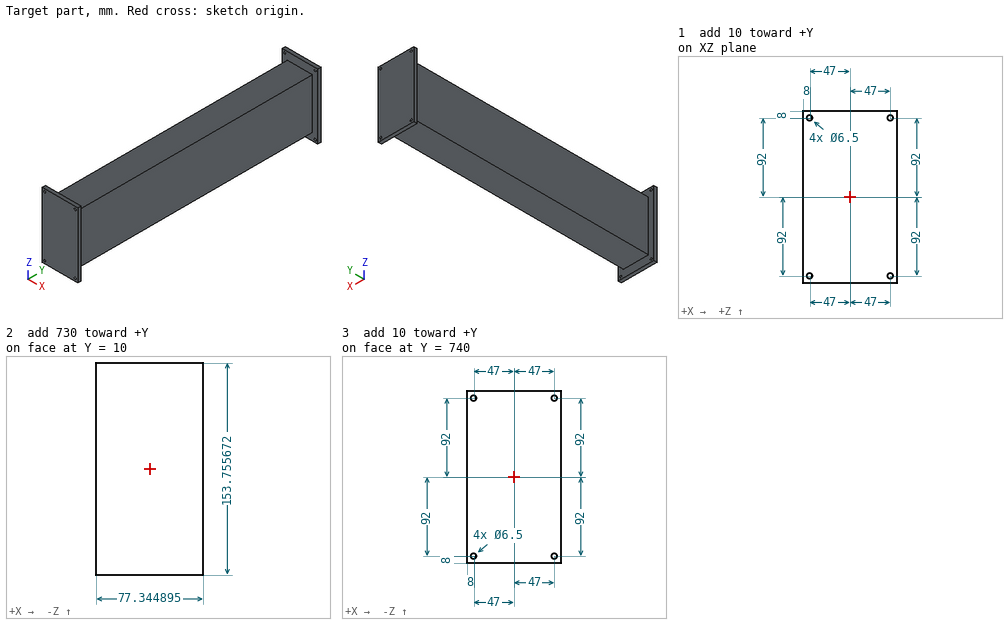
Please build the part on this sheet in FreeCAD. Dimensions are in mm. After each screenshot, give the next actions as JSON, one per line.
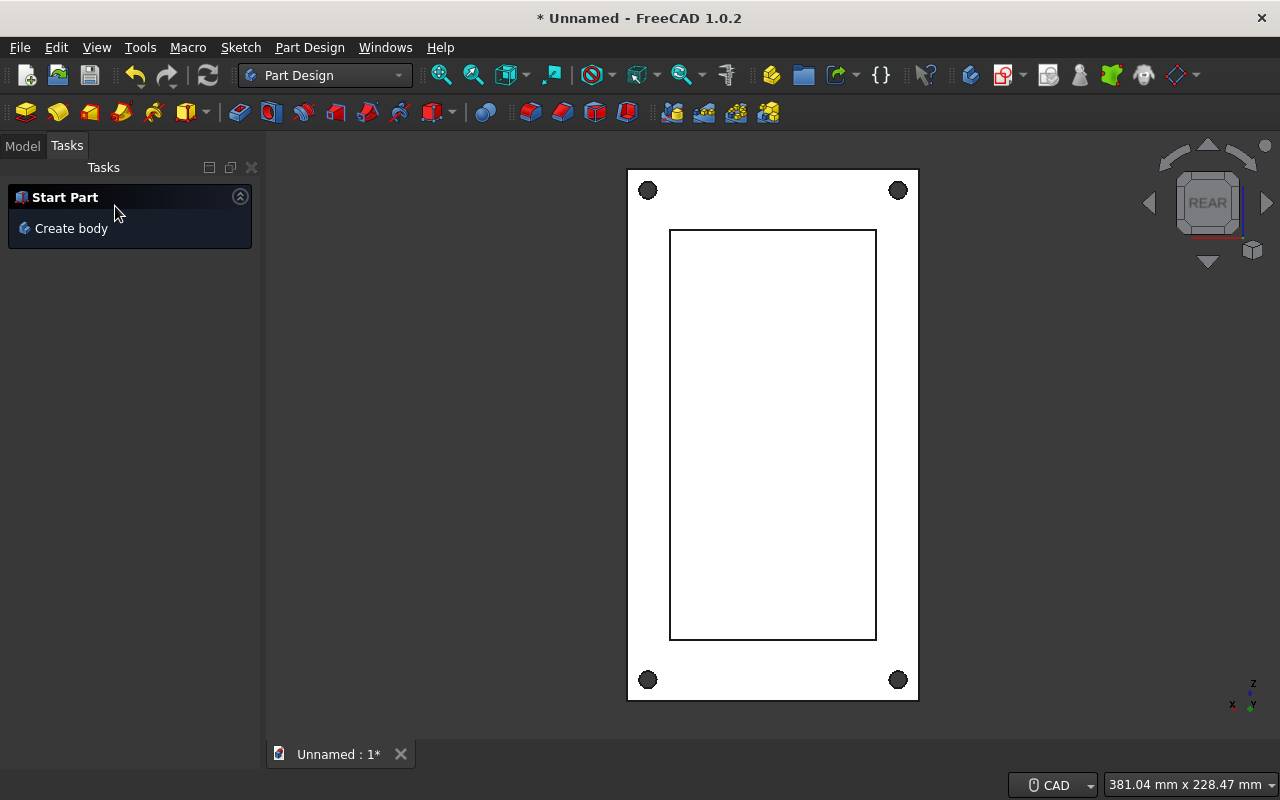
{"action": "left_click", "coordinate": [773, 376]}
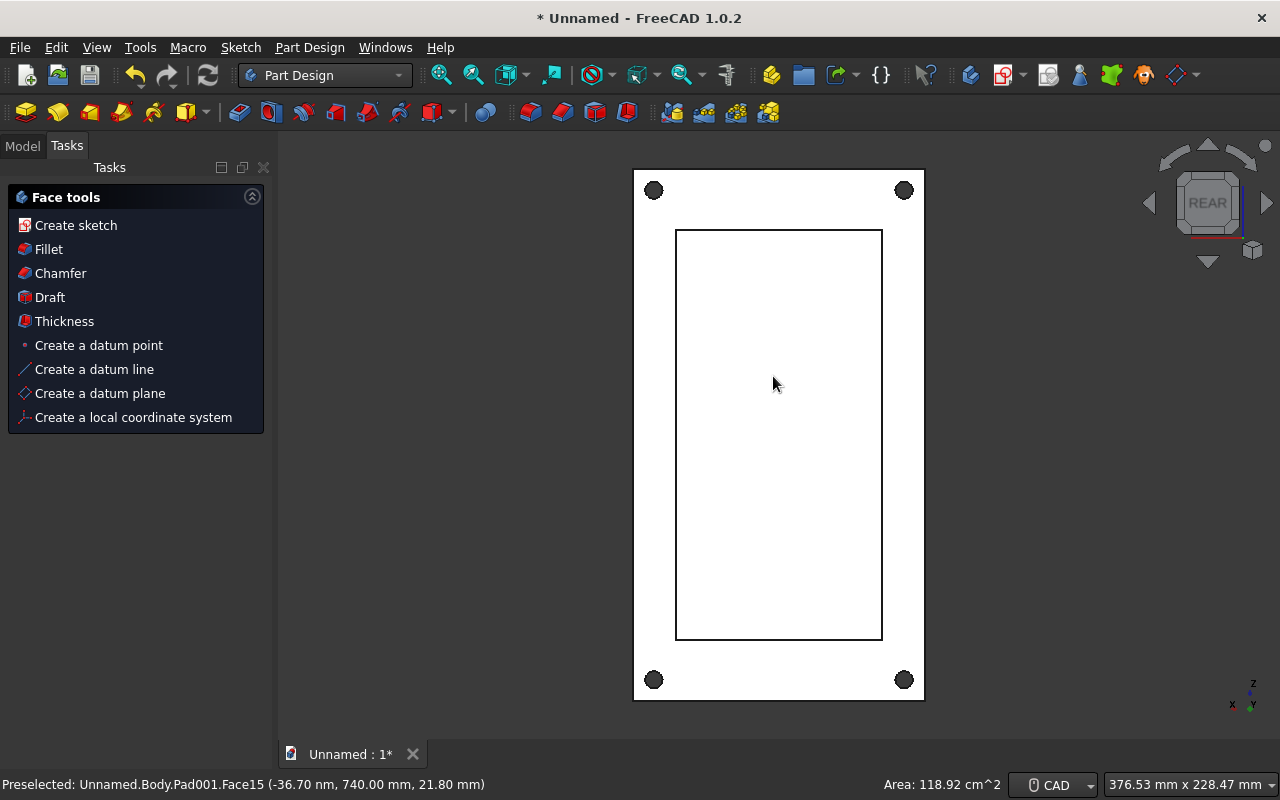
{"action": "left_click", "coordinate": [1004, 76]}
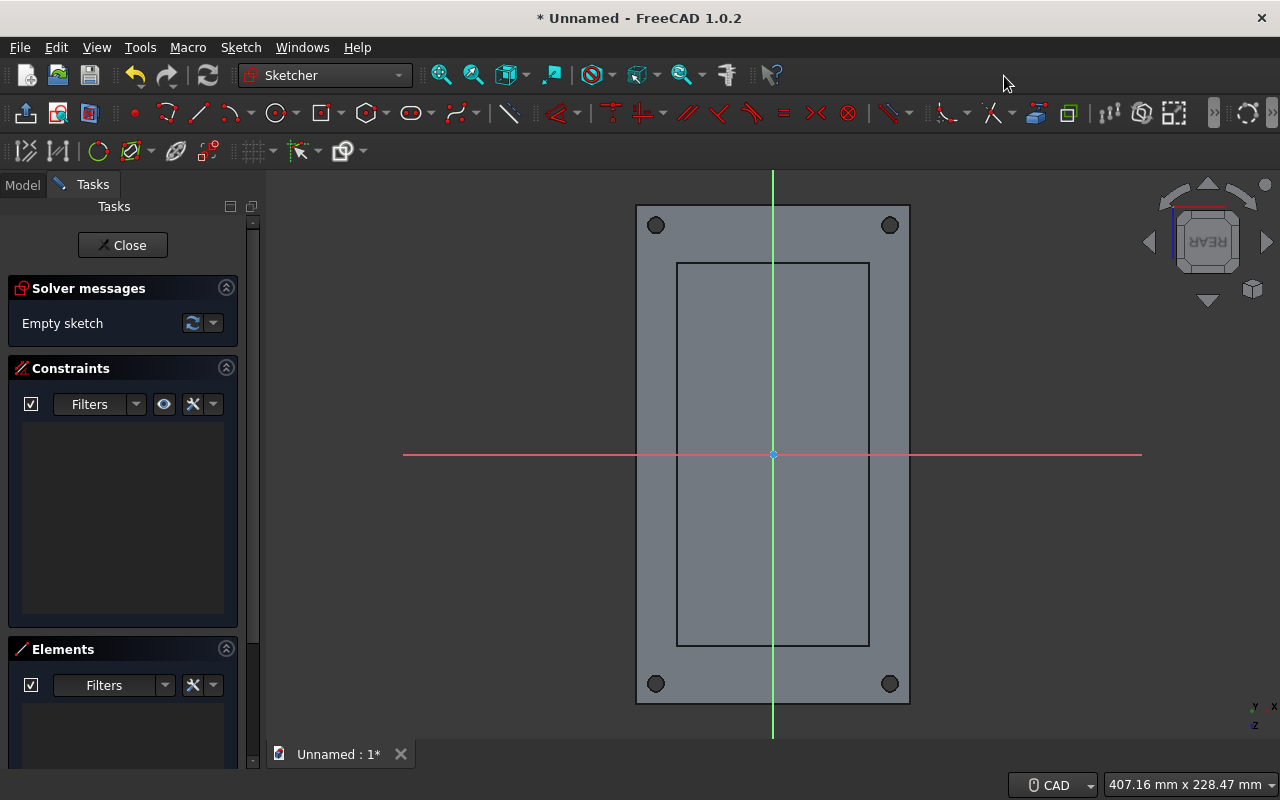
{"action": "scroll", "coordinate": [565, 455], "scroll_direction": "down", "scroll_amount": 2}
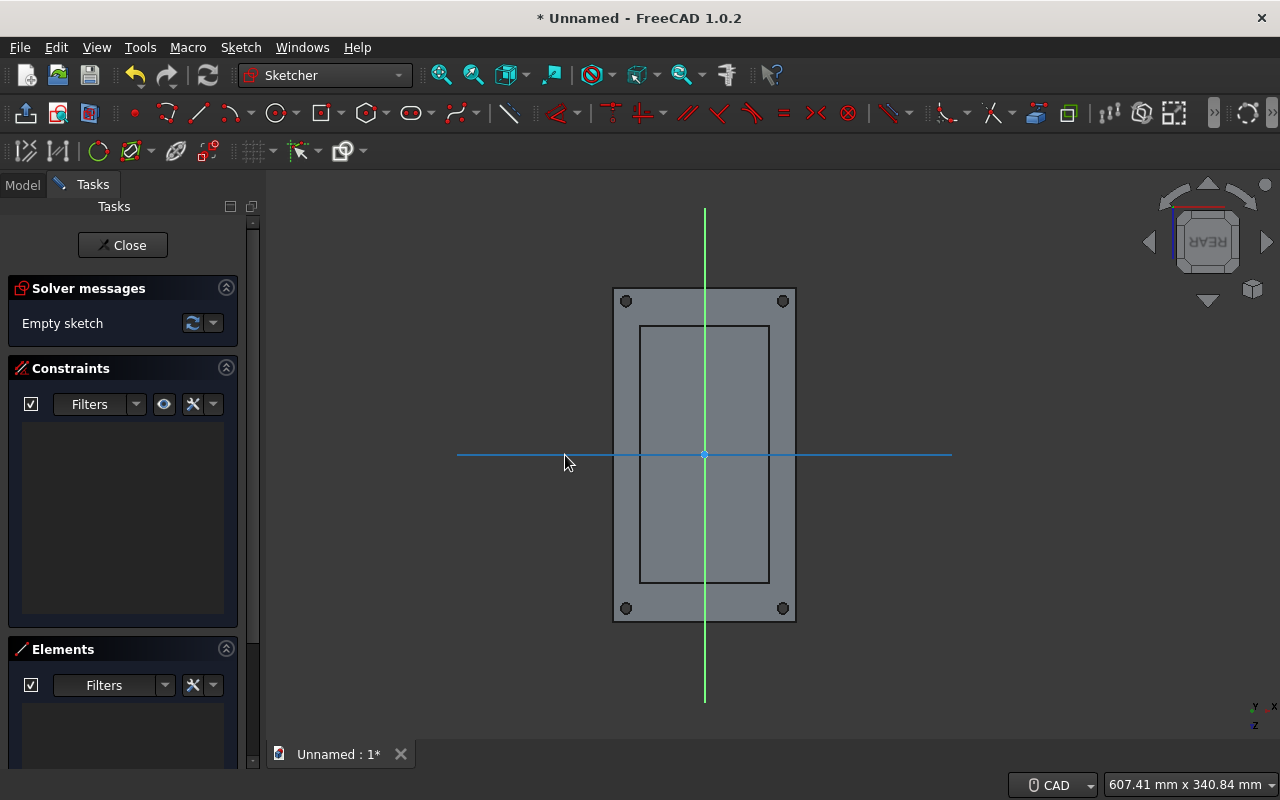
{"action": "left_click", "coordinate": [322, 114]}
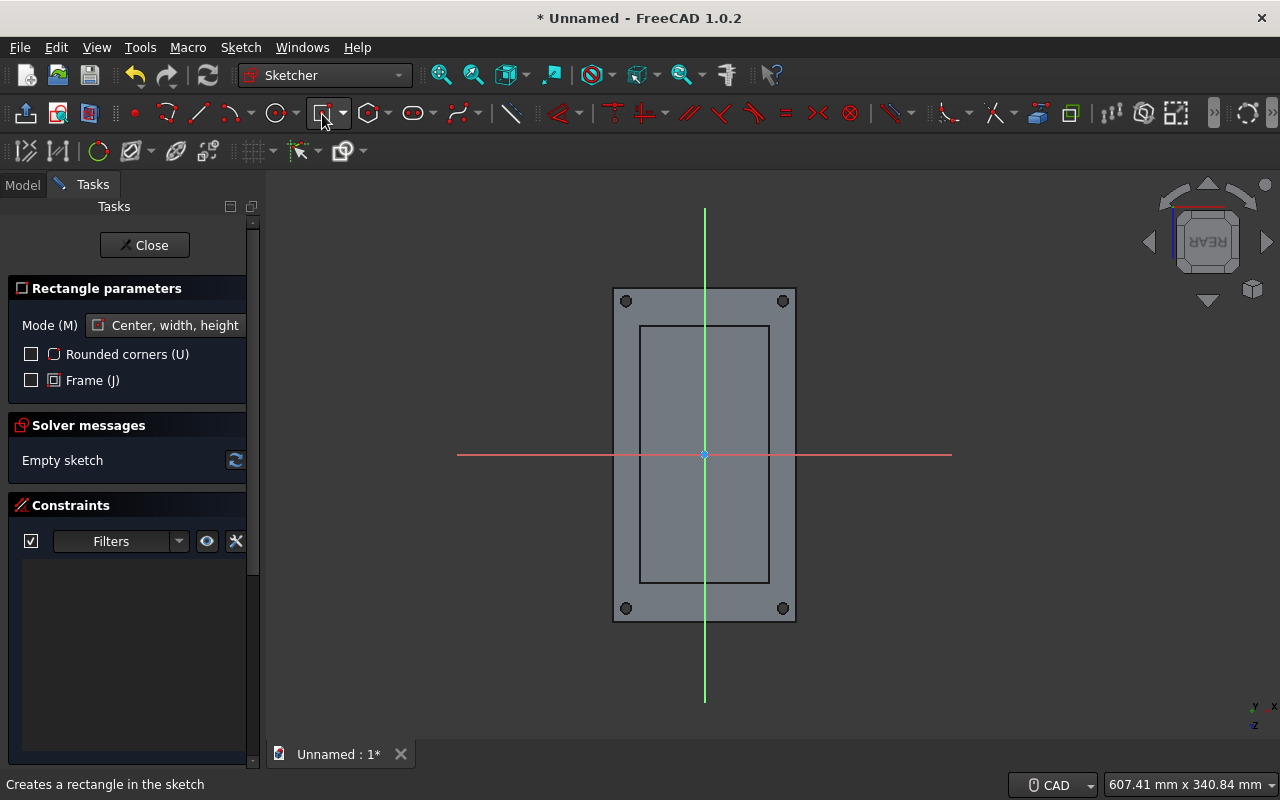
{"action": "left_click", "coordinate": [705, 455]}
{"action": "left_click", "coordinate": [796, 288]}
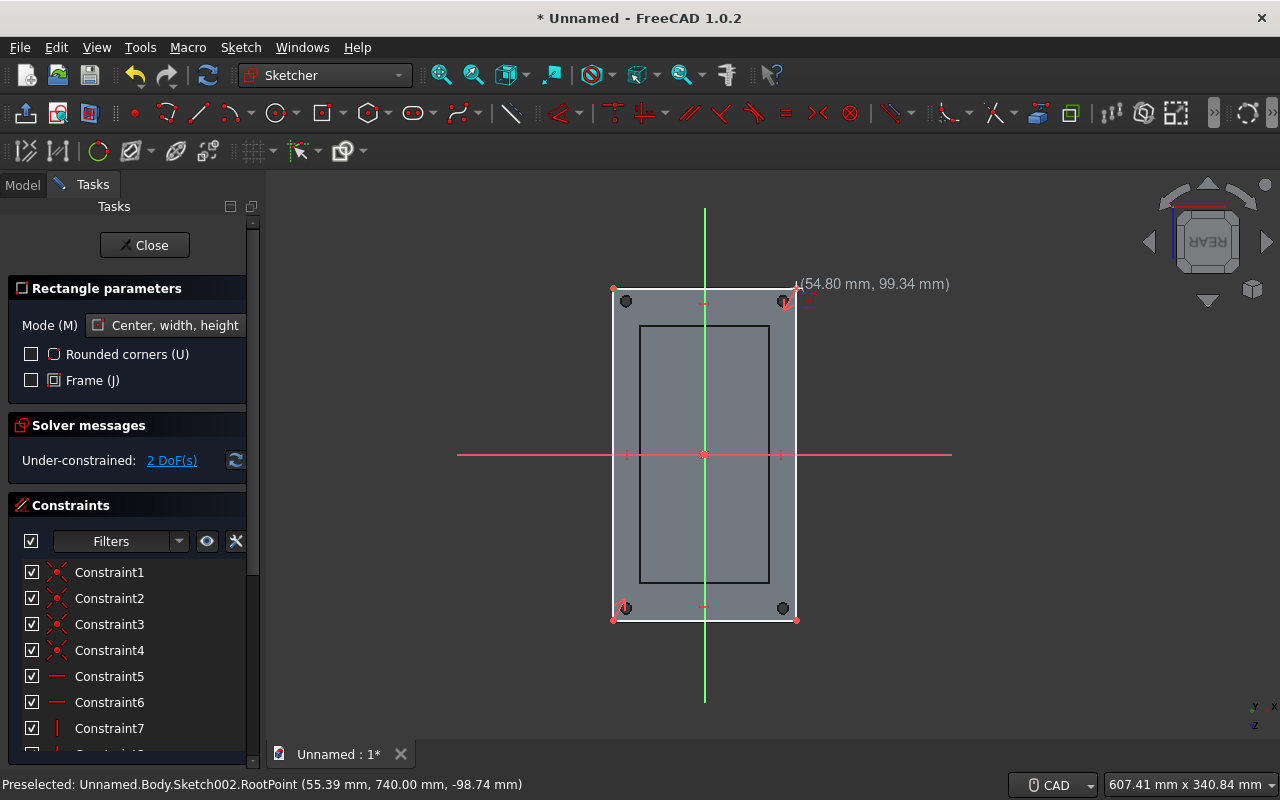
{"action": "left_click", "coordinate": [276, 114]}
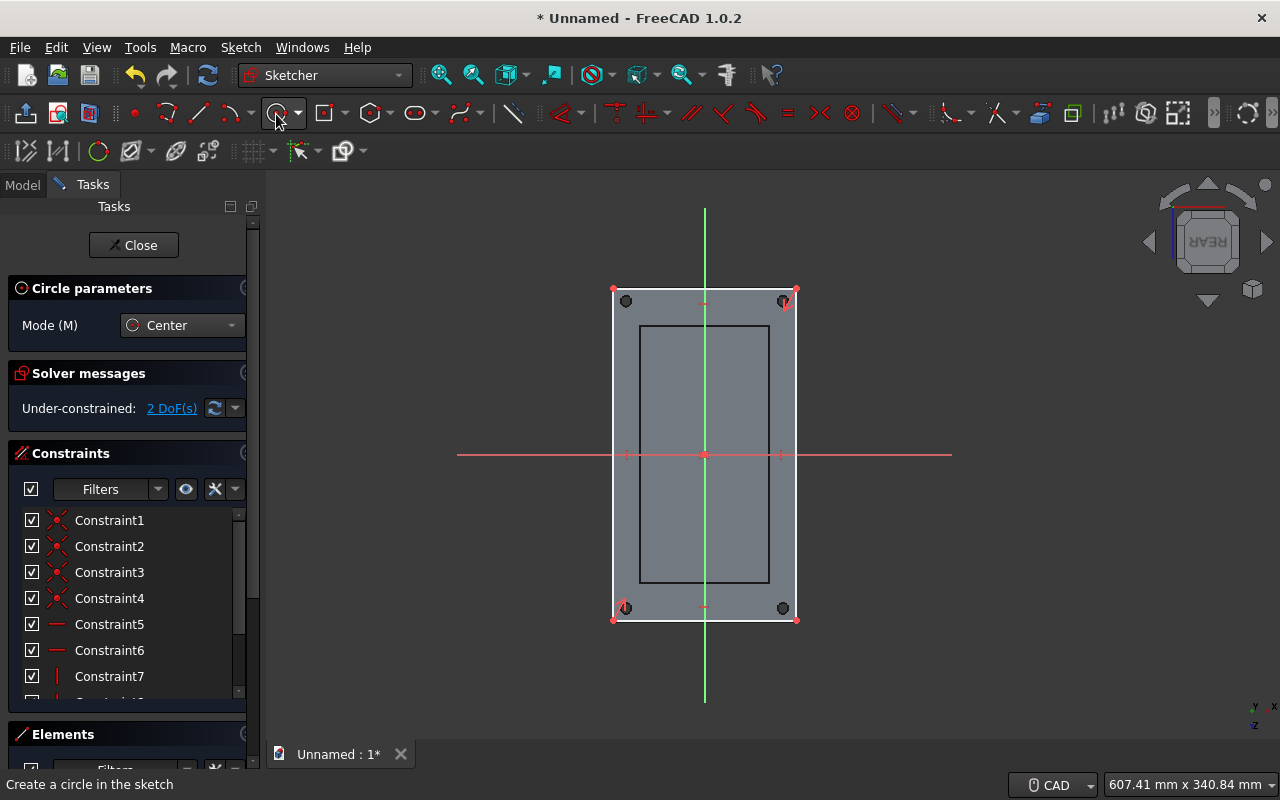
{"action": "scroll", "coordinate": [626, 608], "scroll_direction": "up", "scroll_amount": 8}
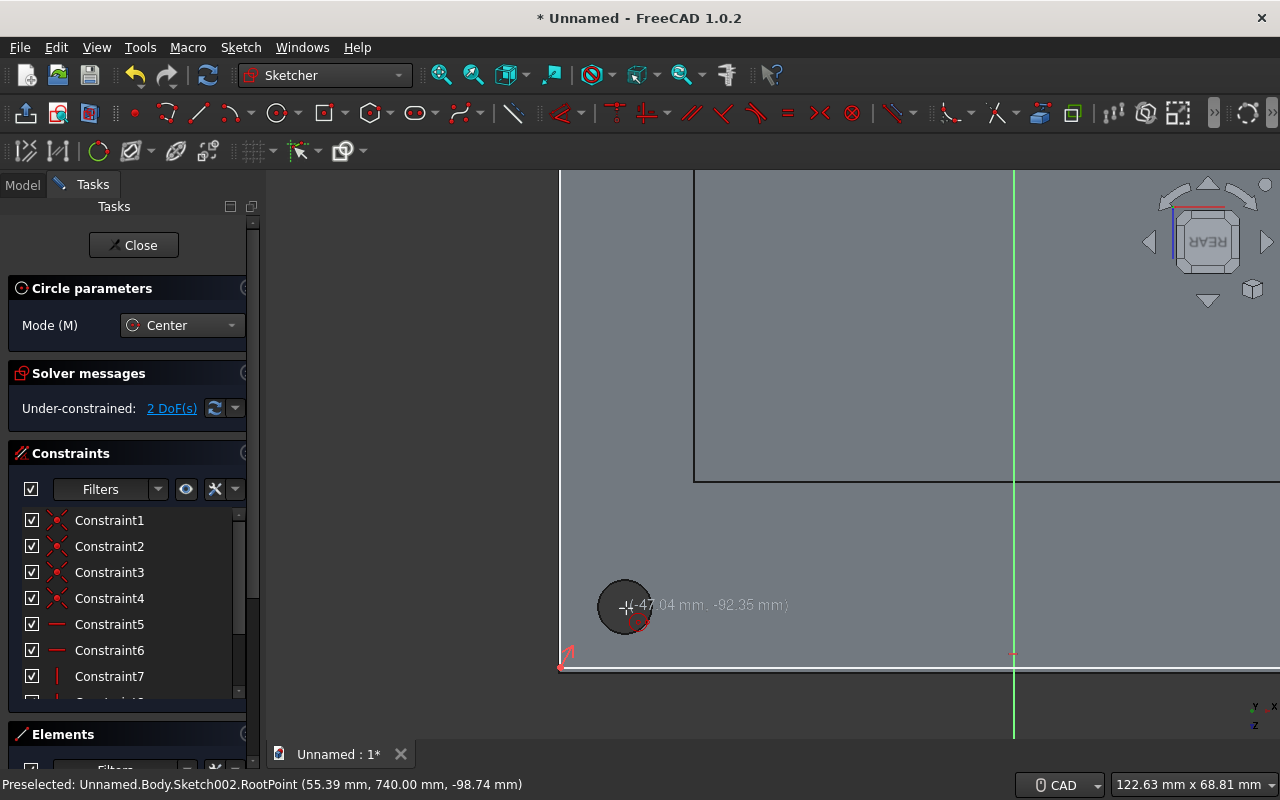
{"action": "scroll", "coordinate": [626, 608], "scroll_direction": "down", "scroll_amount": 8}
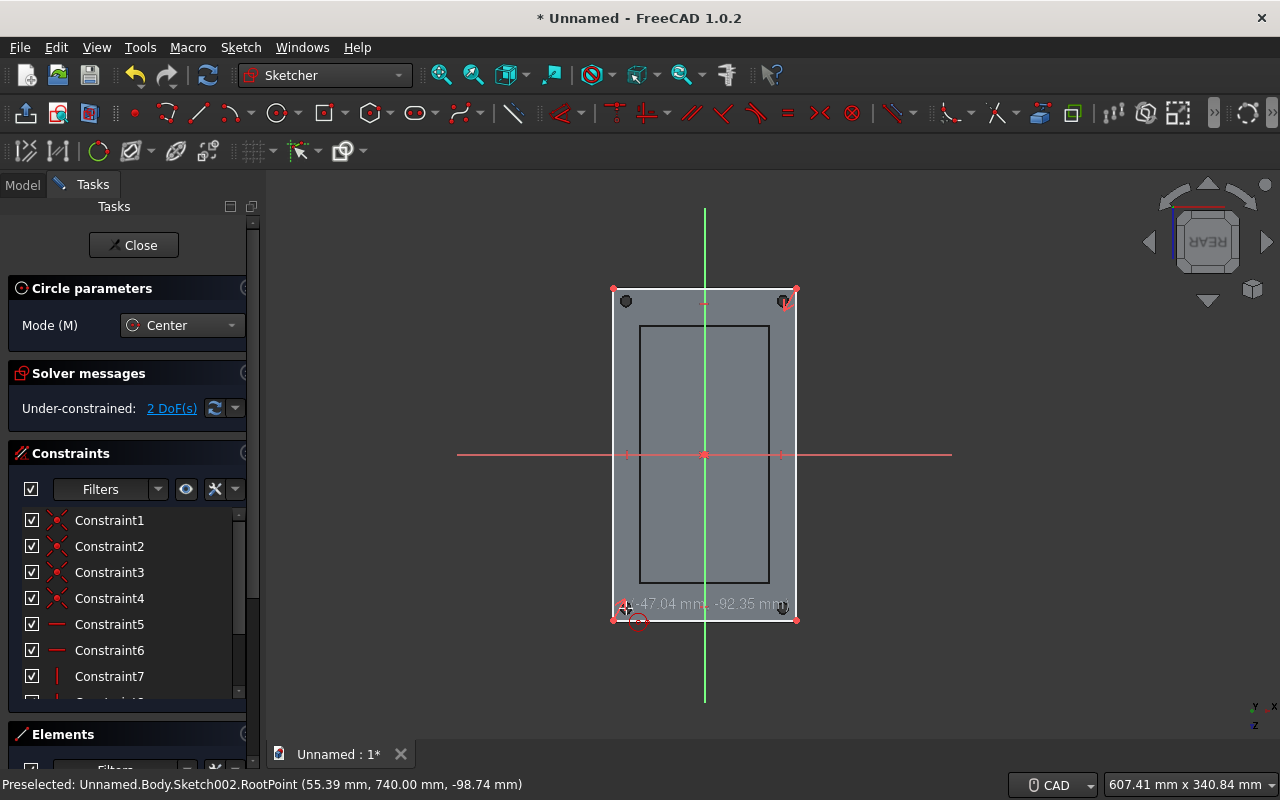
{"action": "left_click", "coordinate": [626, 608]}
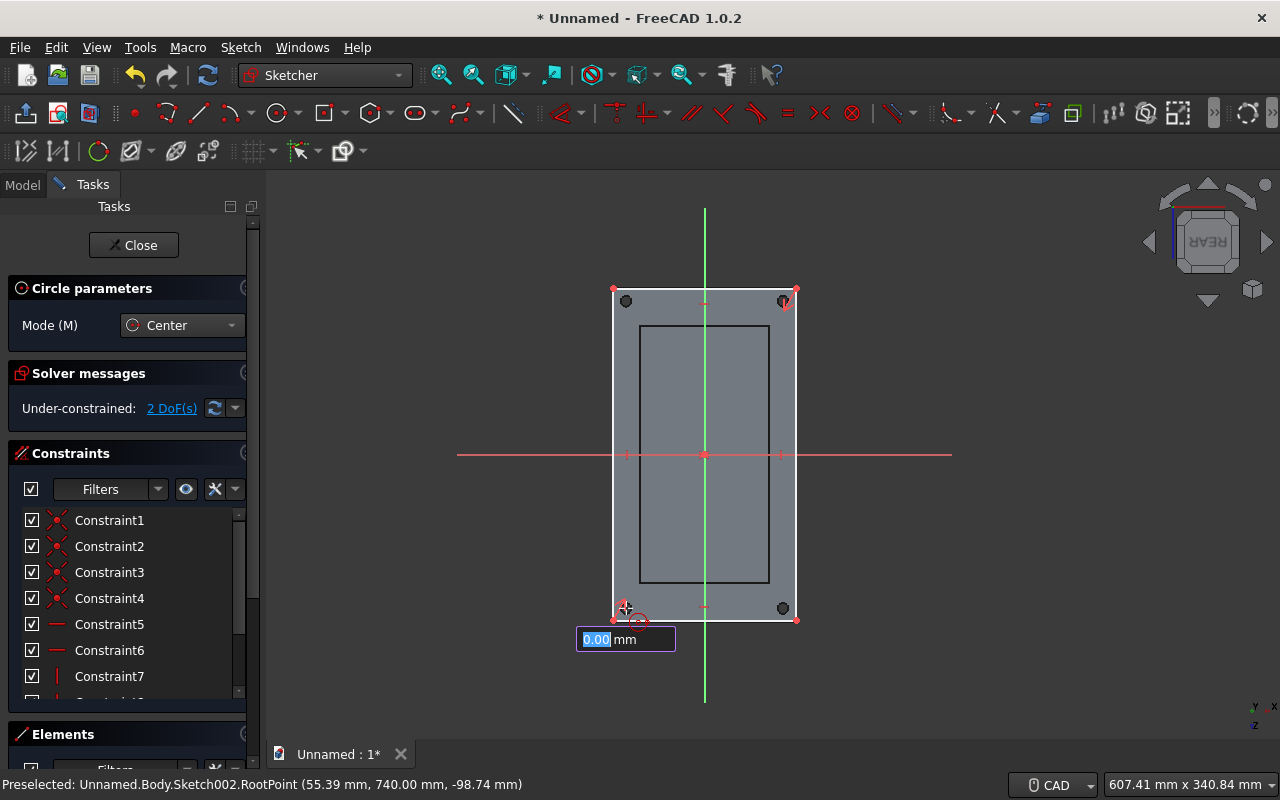
{"action": "scroll", "coordinate": [630, 605], "scroll_direction": "up", "scroll_amount": 6}